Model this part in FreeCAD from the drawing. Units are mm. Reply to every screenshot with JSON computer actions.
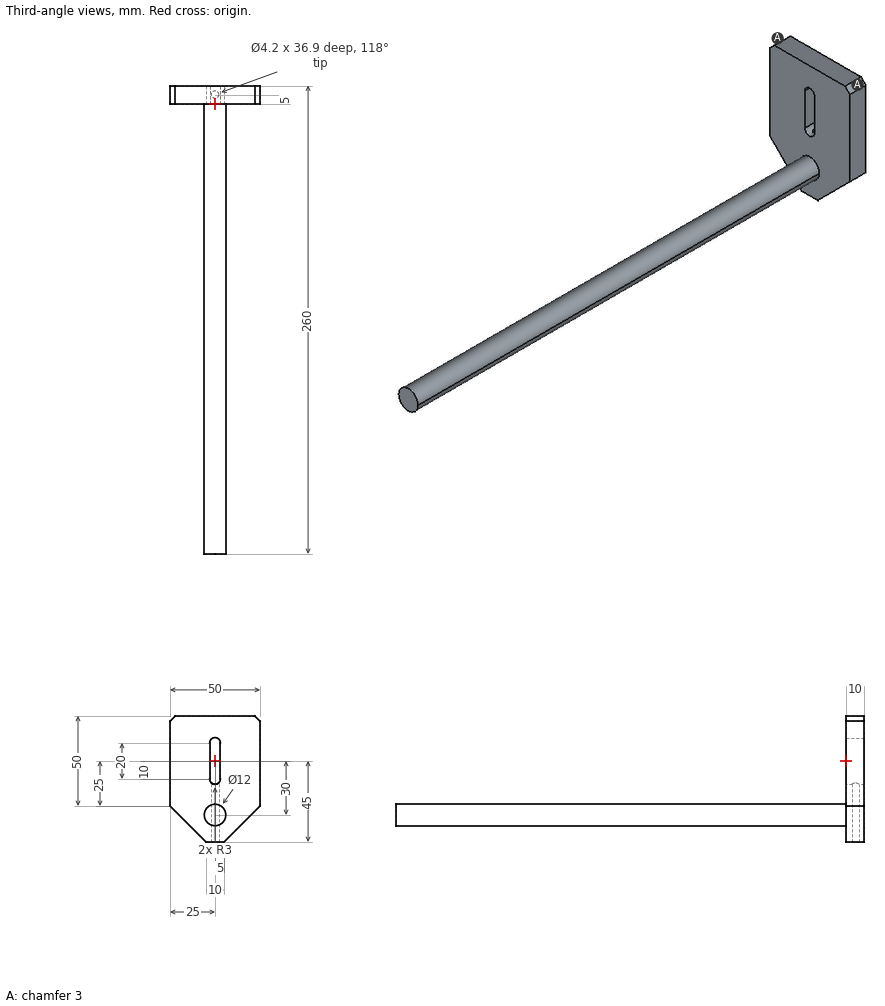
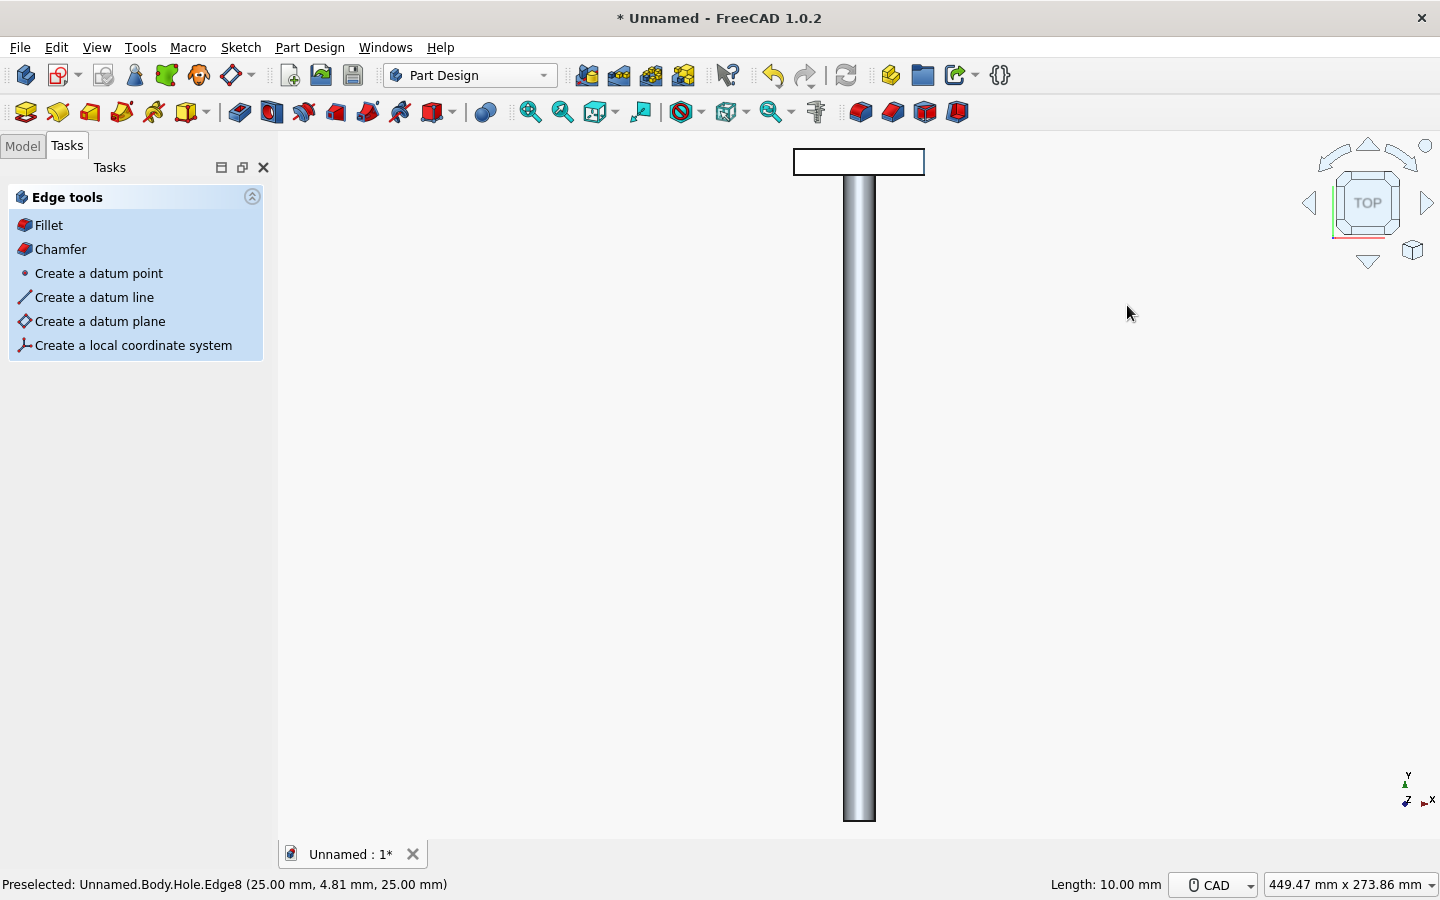
{"action": "left_click", "coordinate": [794, 161], "text": "ctrl"}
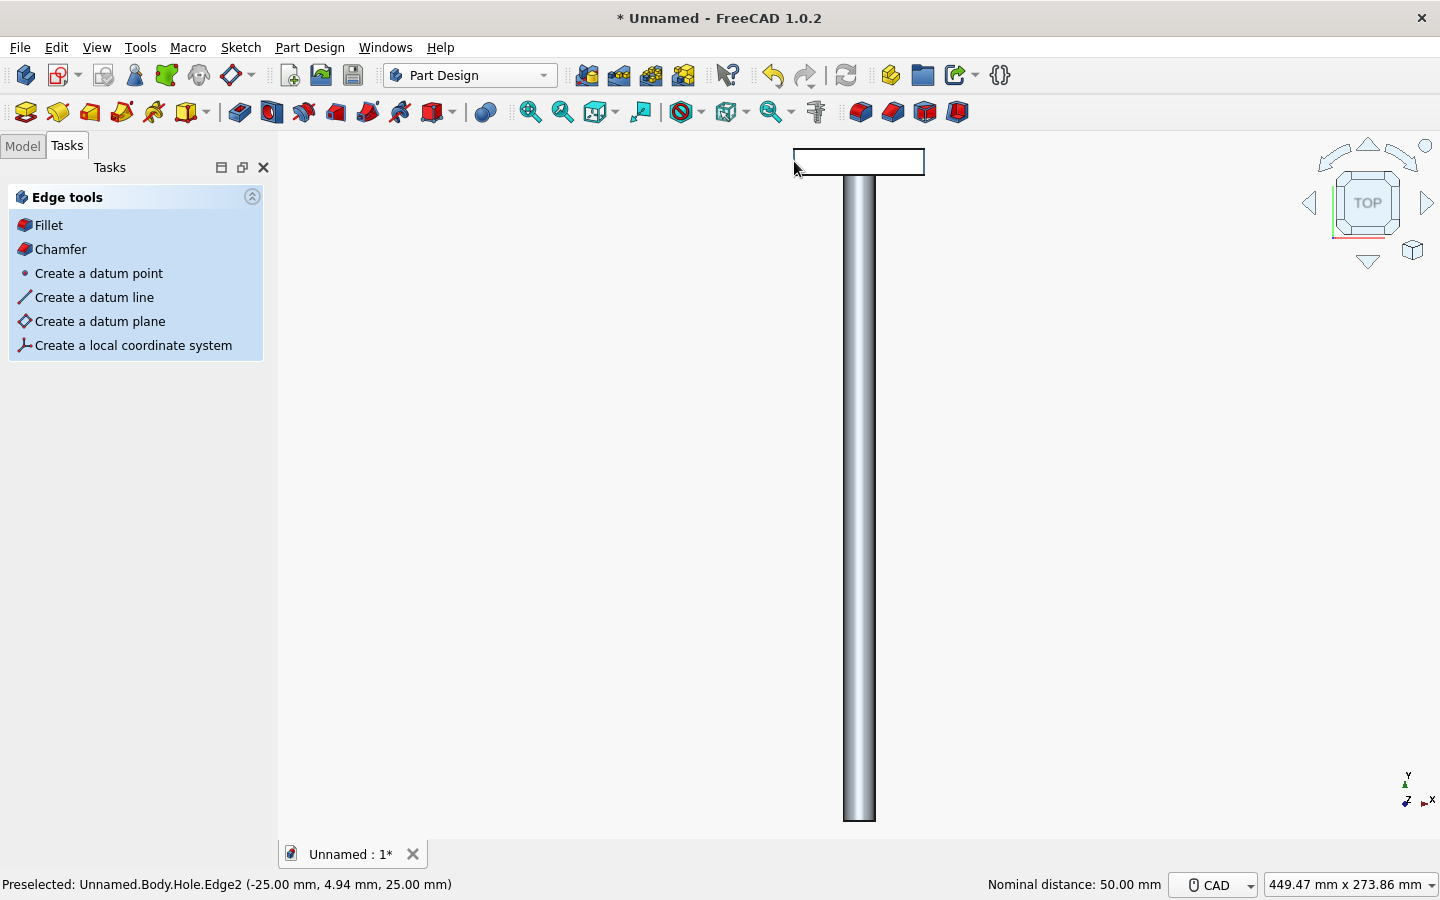
{"action": "left_click", "coordinate": [894, 112]}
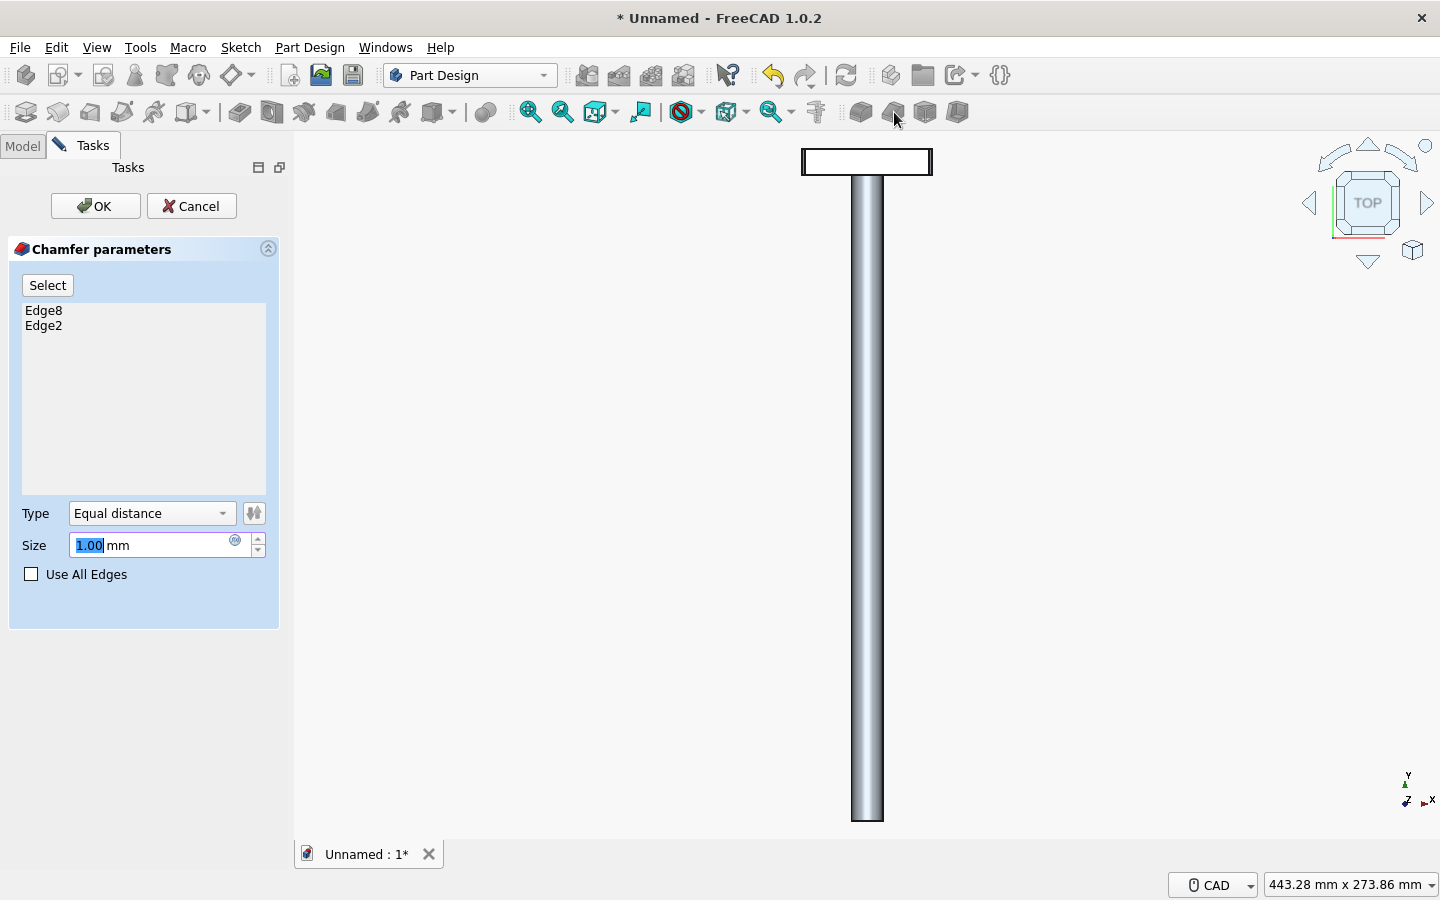
{"action": "type", "text": "3"}
{"action": "key", "text": "Tab"}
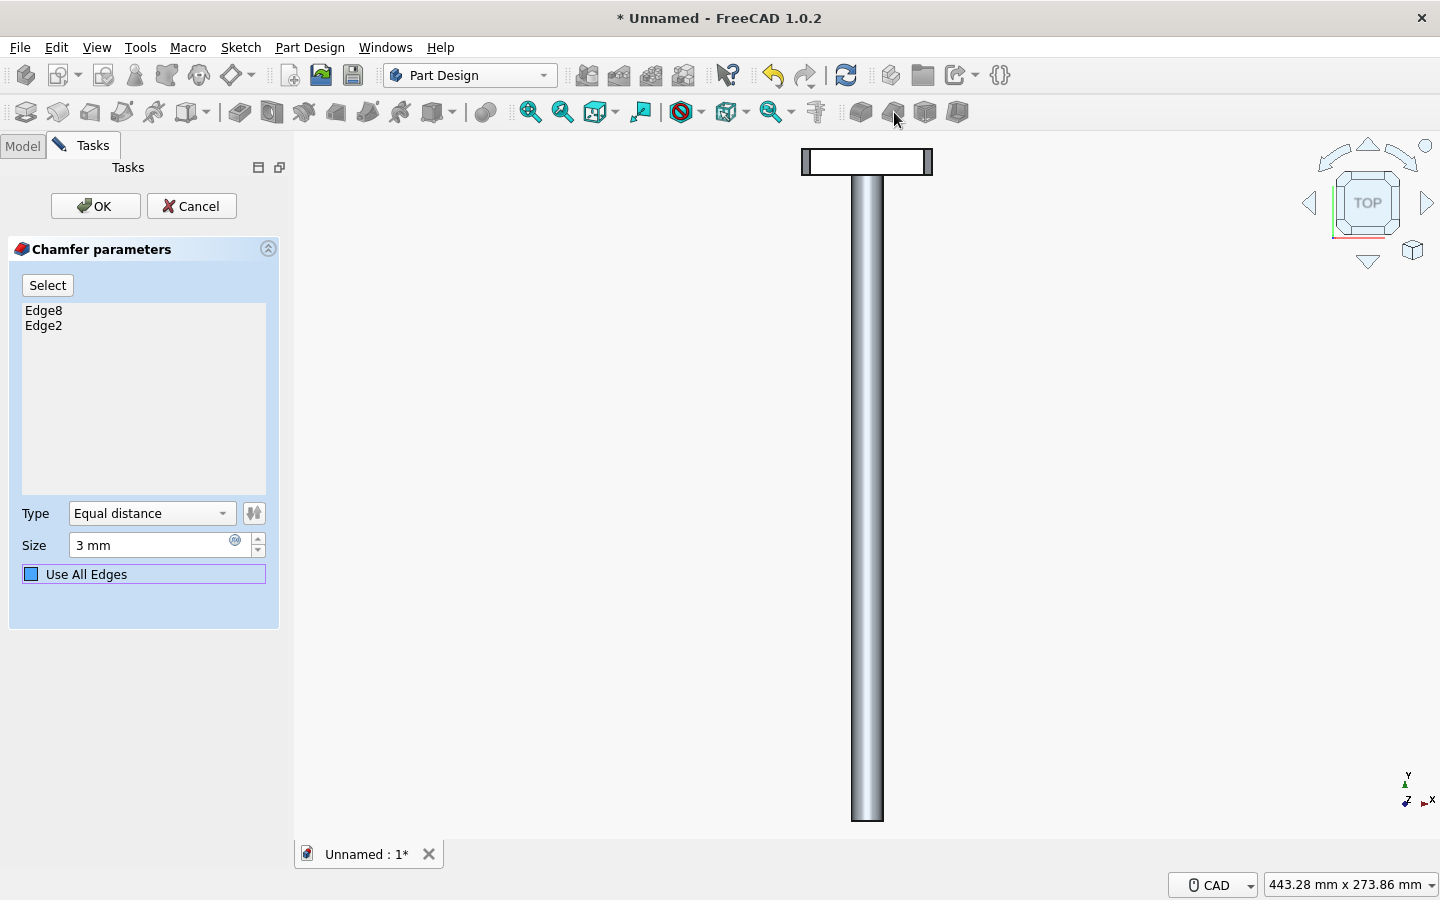
{"action": "left_click", "coordinate": [96, 206]}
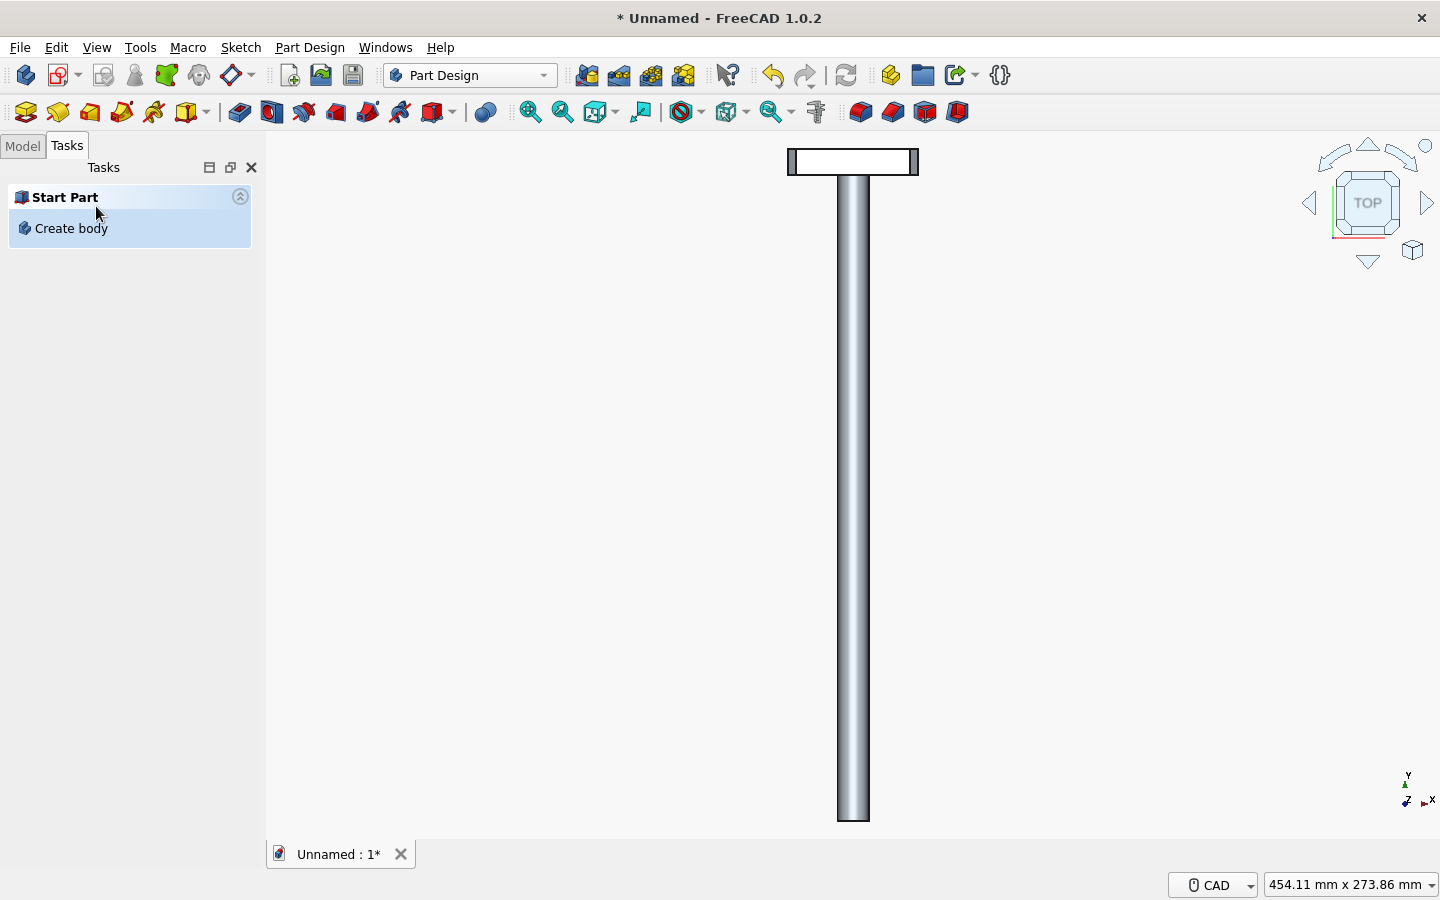
{"action": "key", "text": "0"}